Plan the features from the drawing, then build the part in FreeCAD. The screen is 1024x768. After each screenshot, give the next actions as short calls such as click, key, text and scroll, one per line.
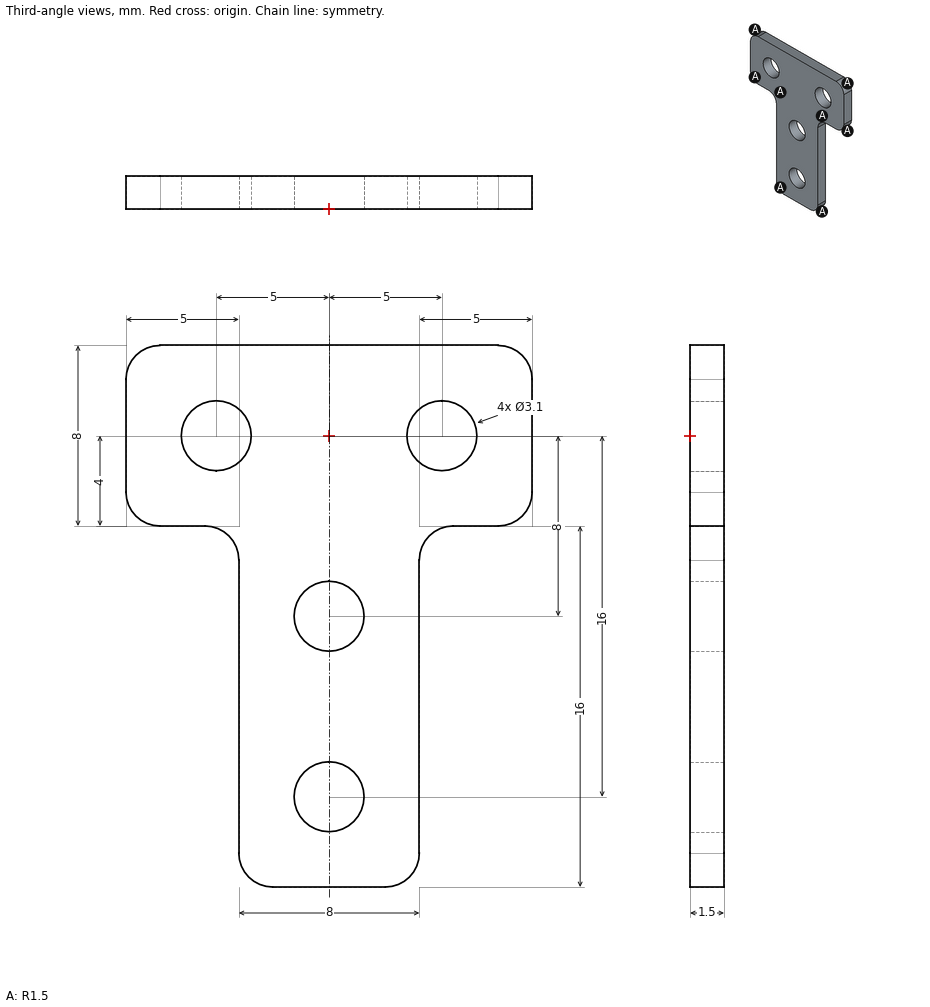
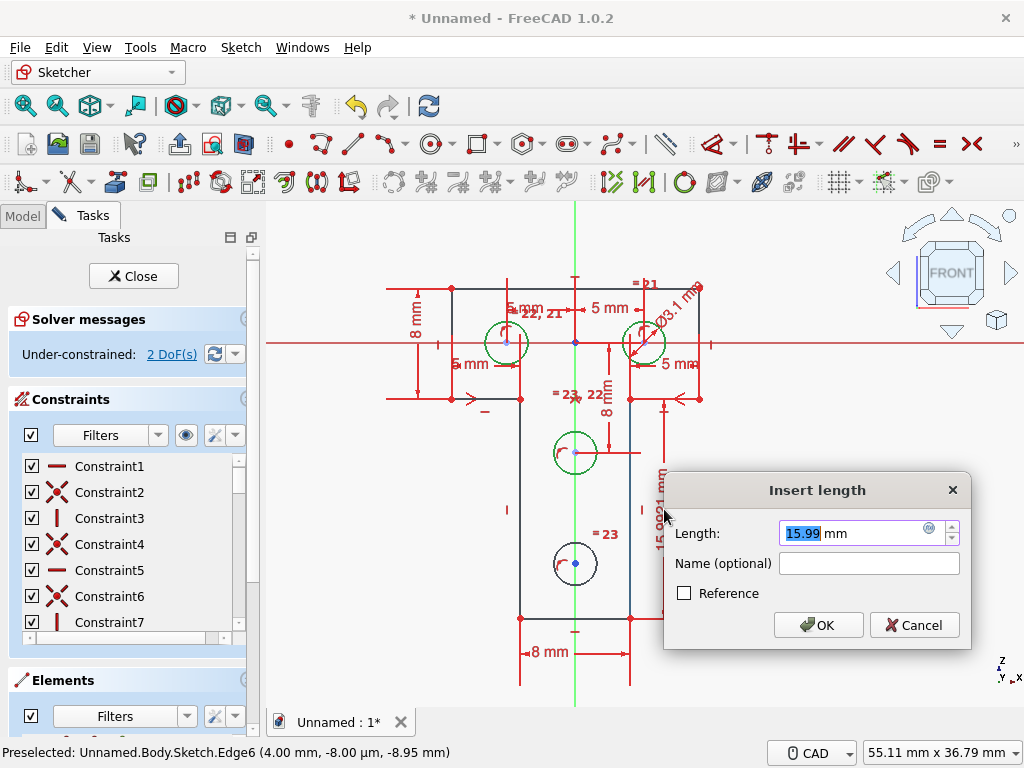
text(16)
key(Return)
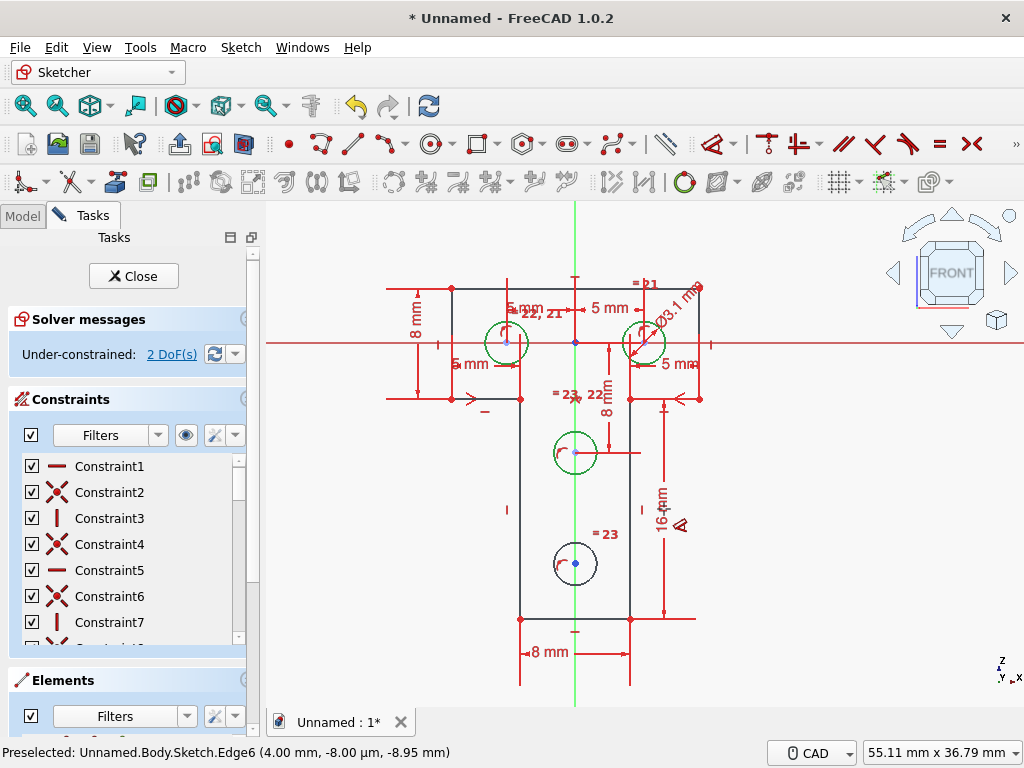
click(520, 399)
click(609, 371)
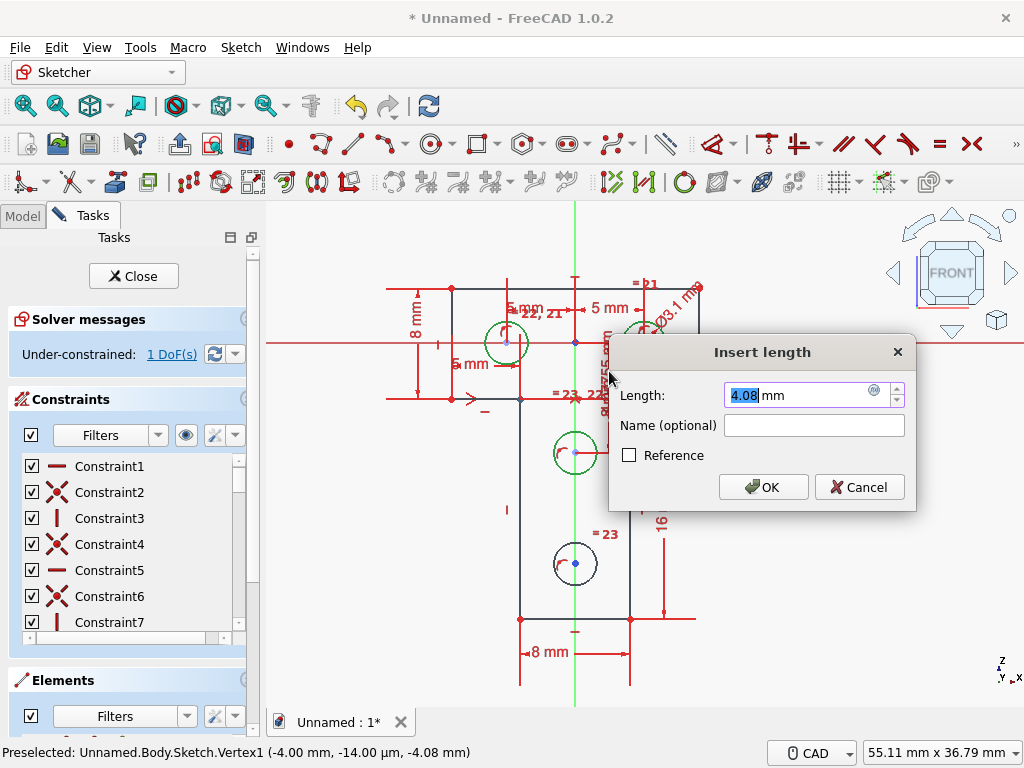
text(4)
key(Return)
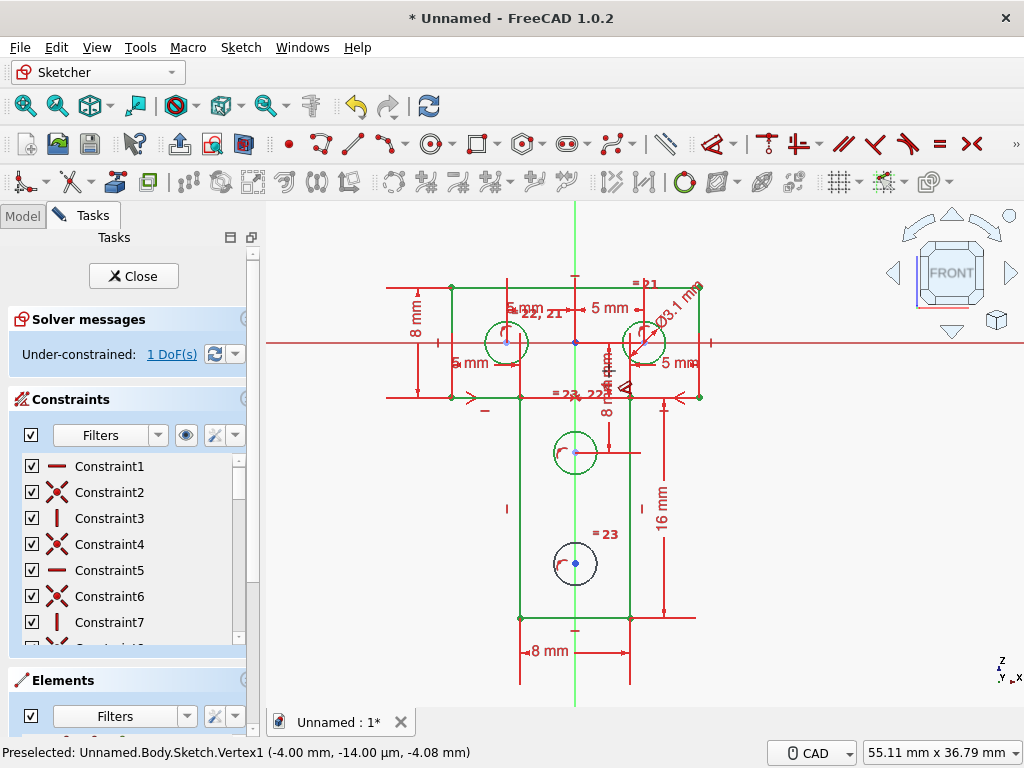
click(575, 564)
click(609, 531)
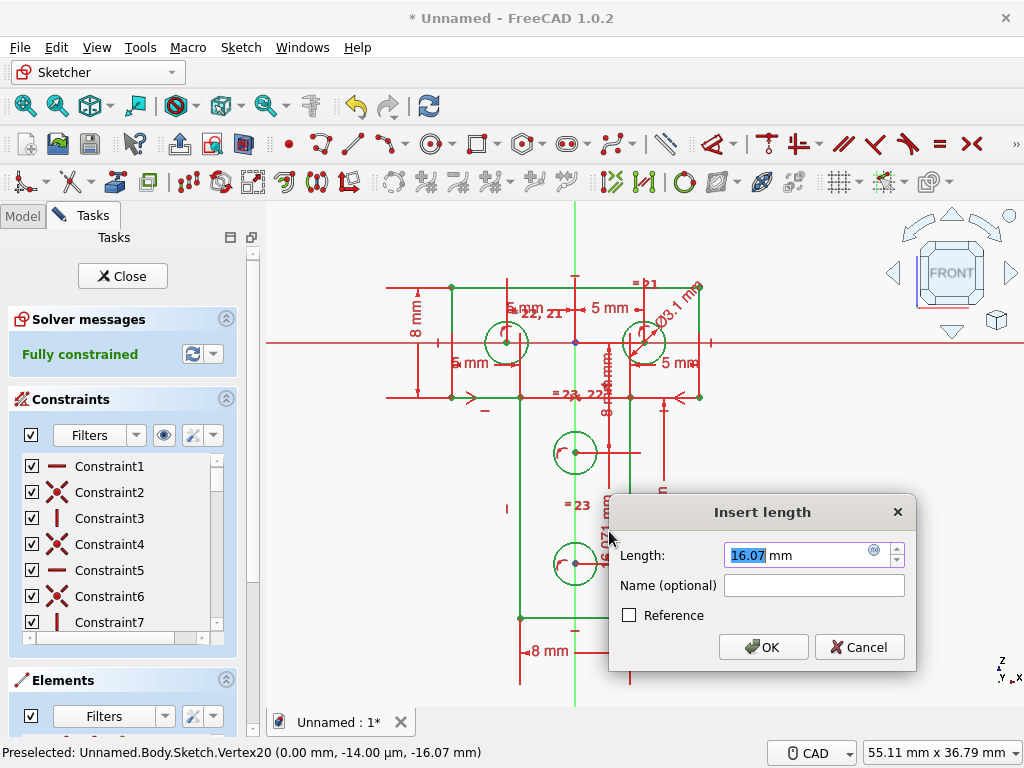
text(16)
key(Return)
key(Escape)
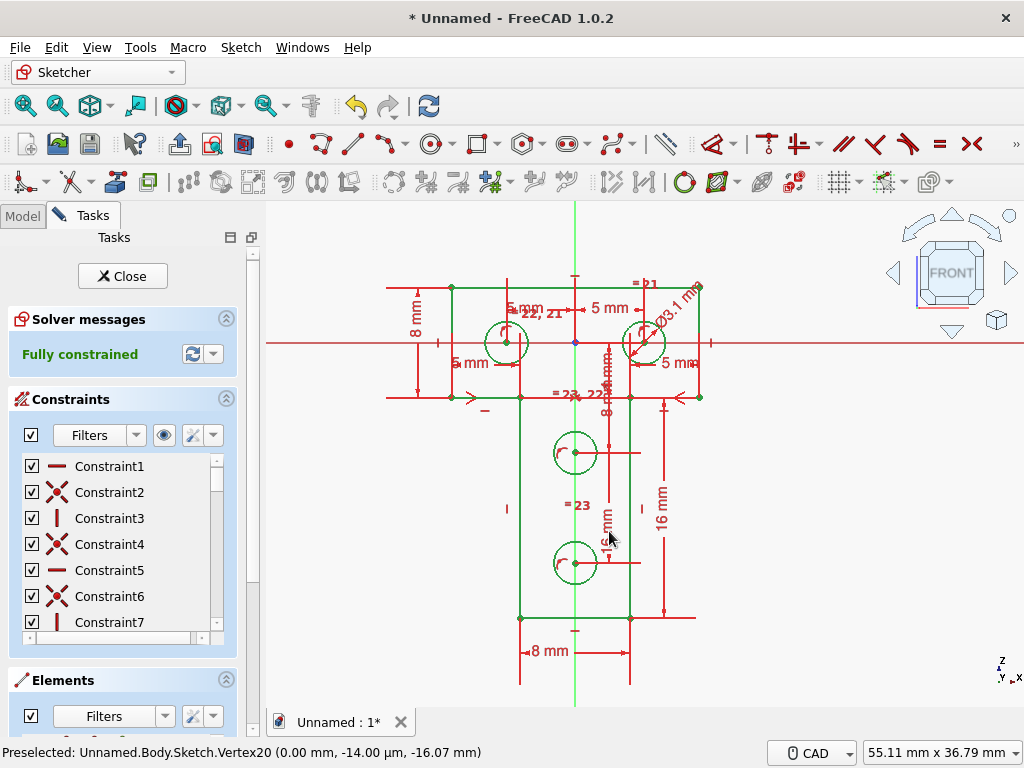
click(123, 276)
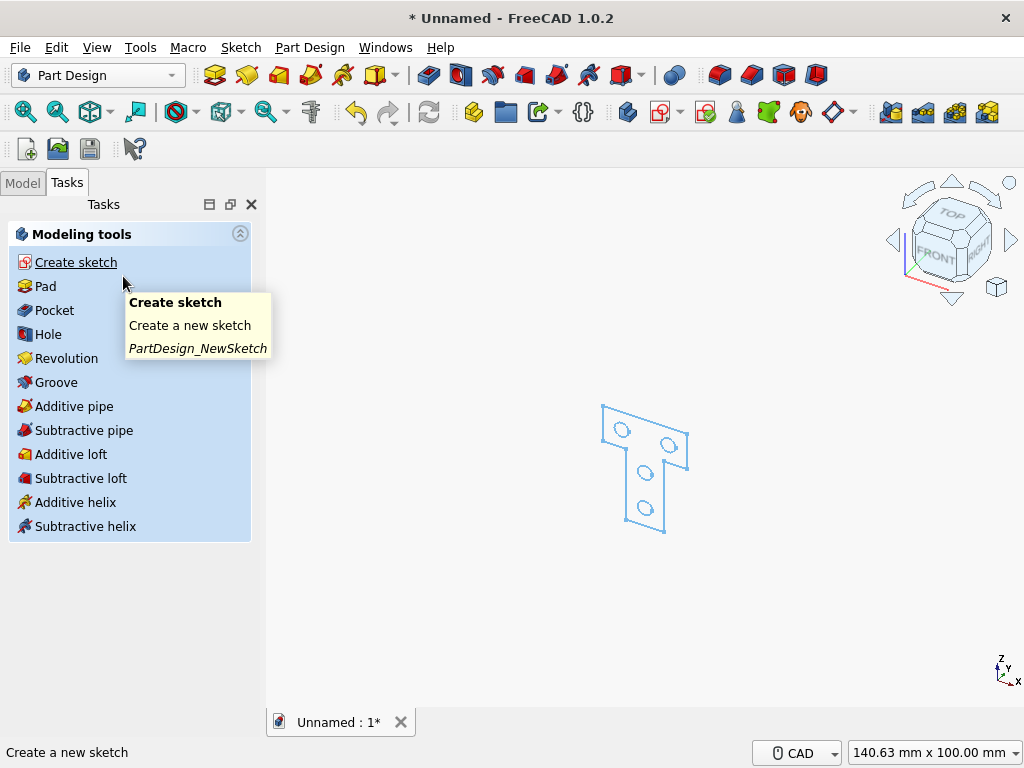
click(216, 76)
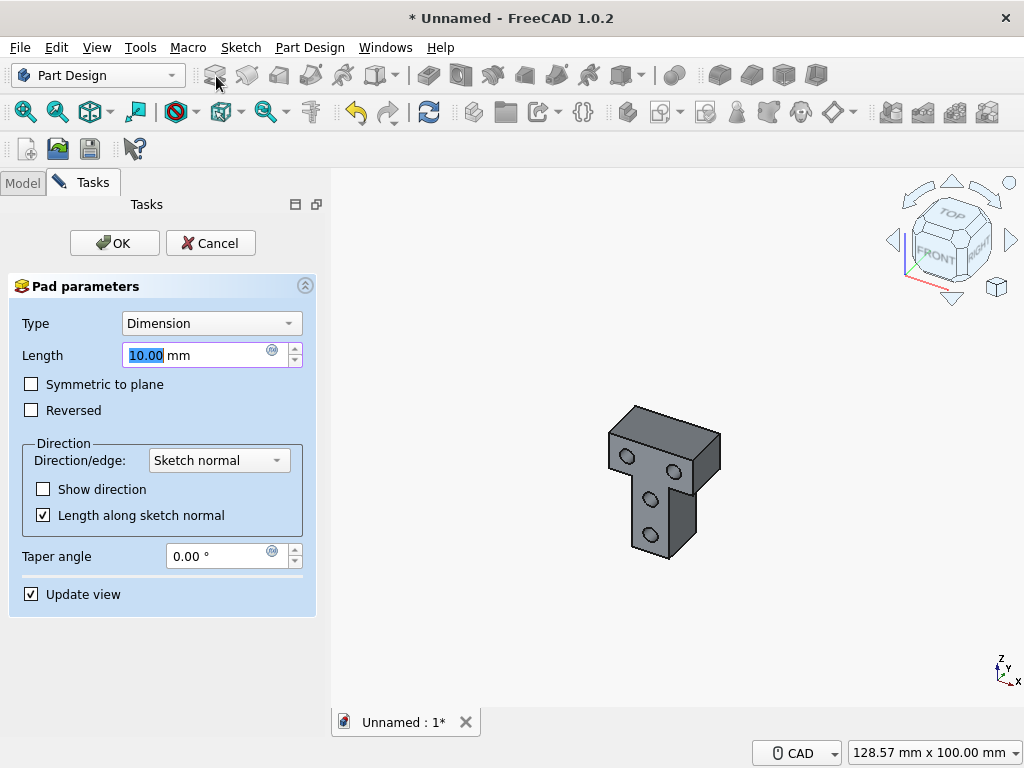
text(1.5)
key(Tab)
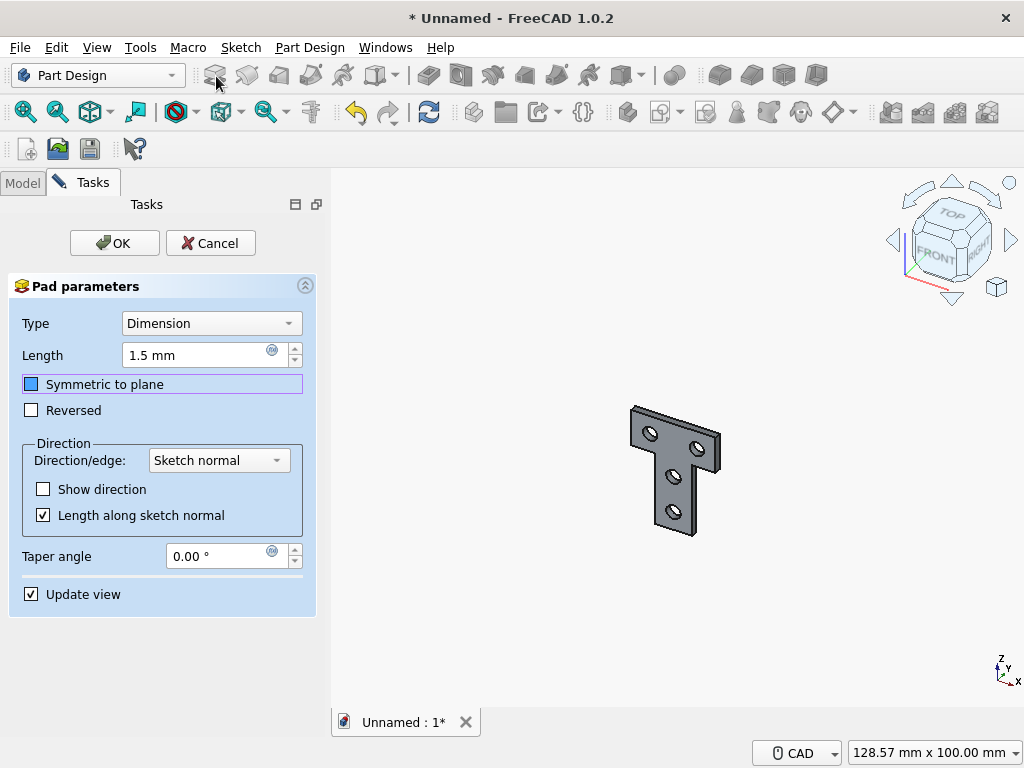
click(30, 410)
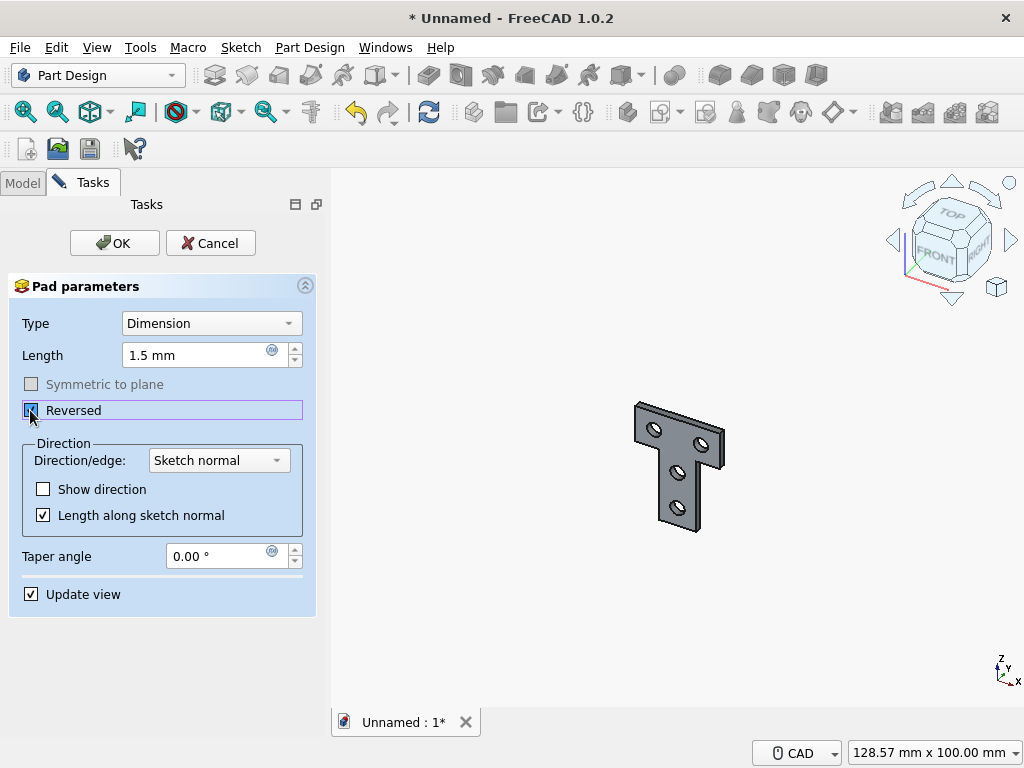
click(115, 243)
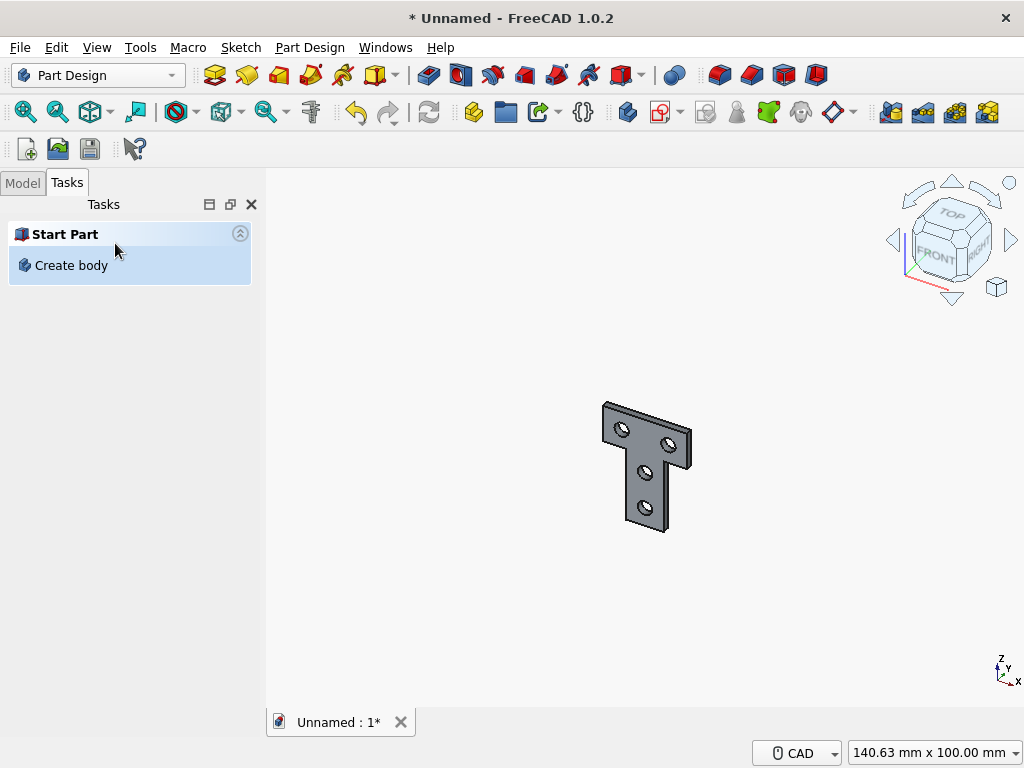
click(26, 112)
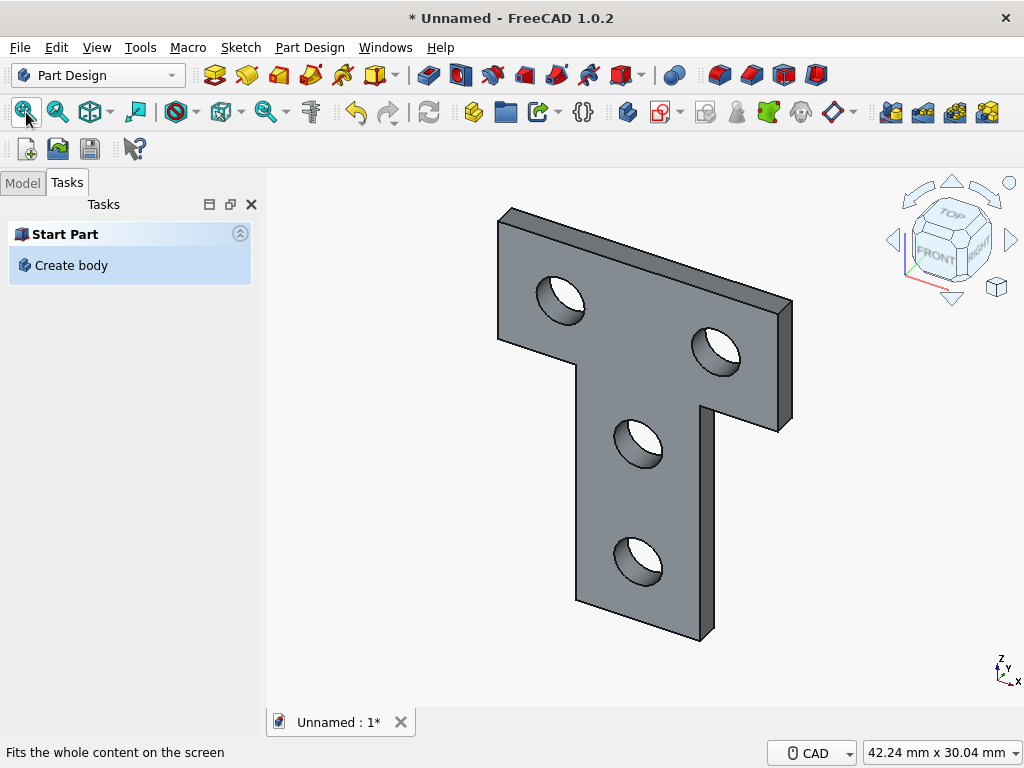
click(785, 306)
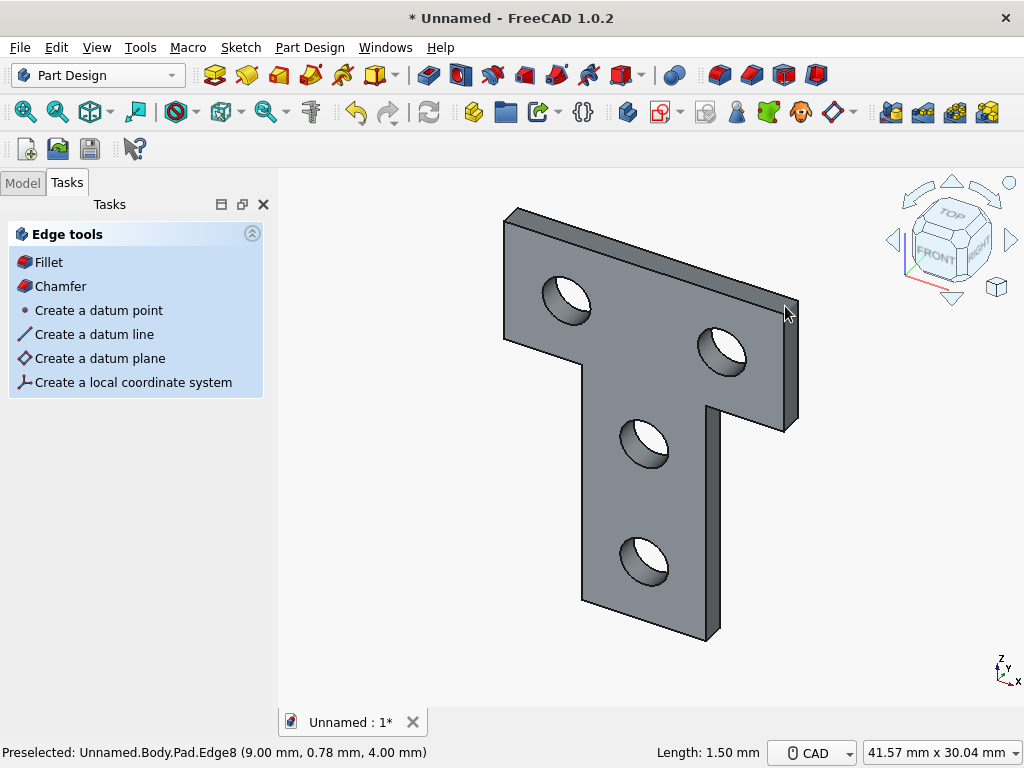
key(0)